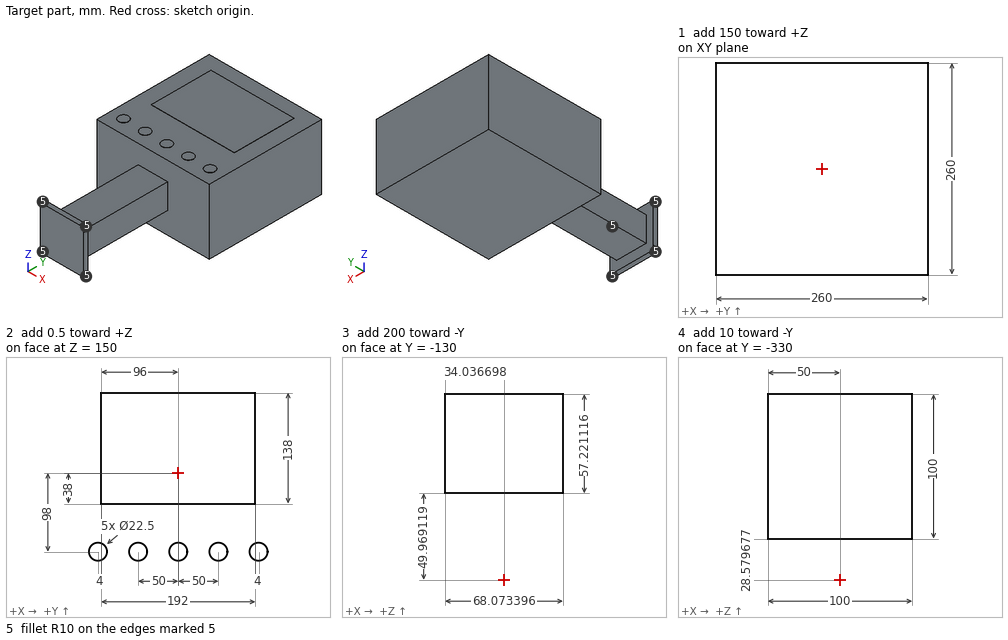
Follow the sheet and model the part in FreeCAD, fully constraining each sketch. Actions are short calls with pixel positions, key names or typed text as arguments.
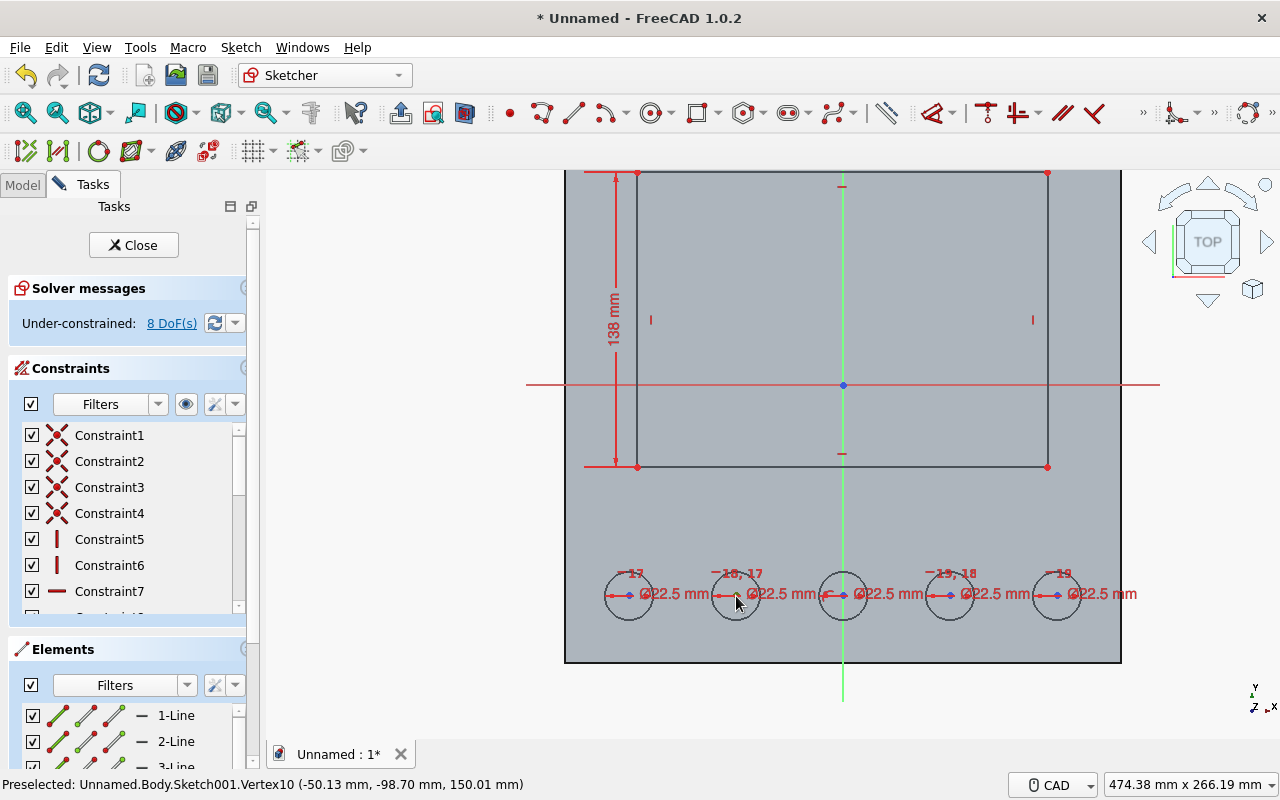
click(843, 596)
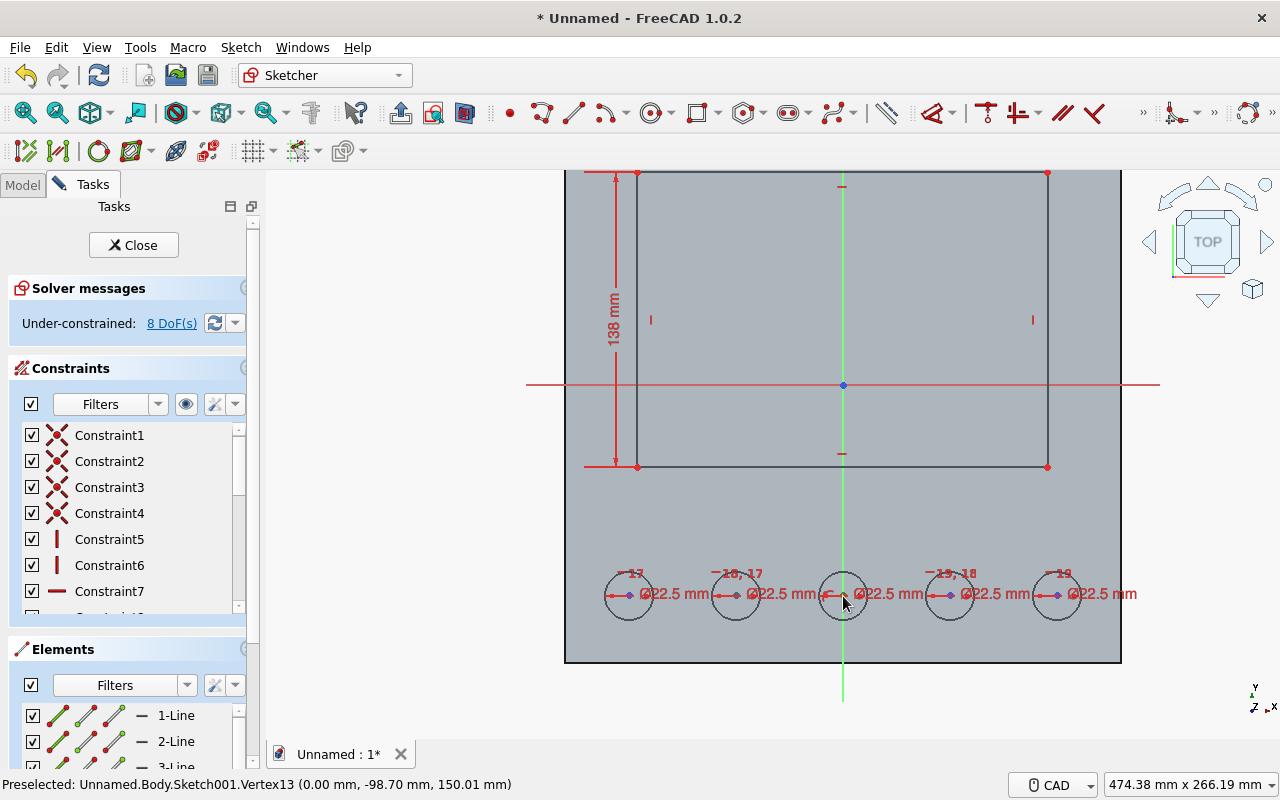
key(h)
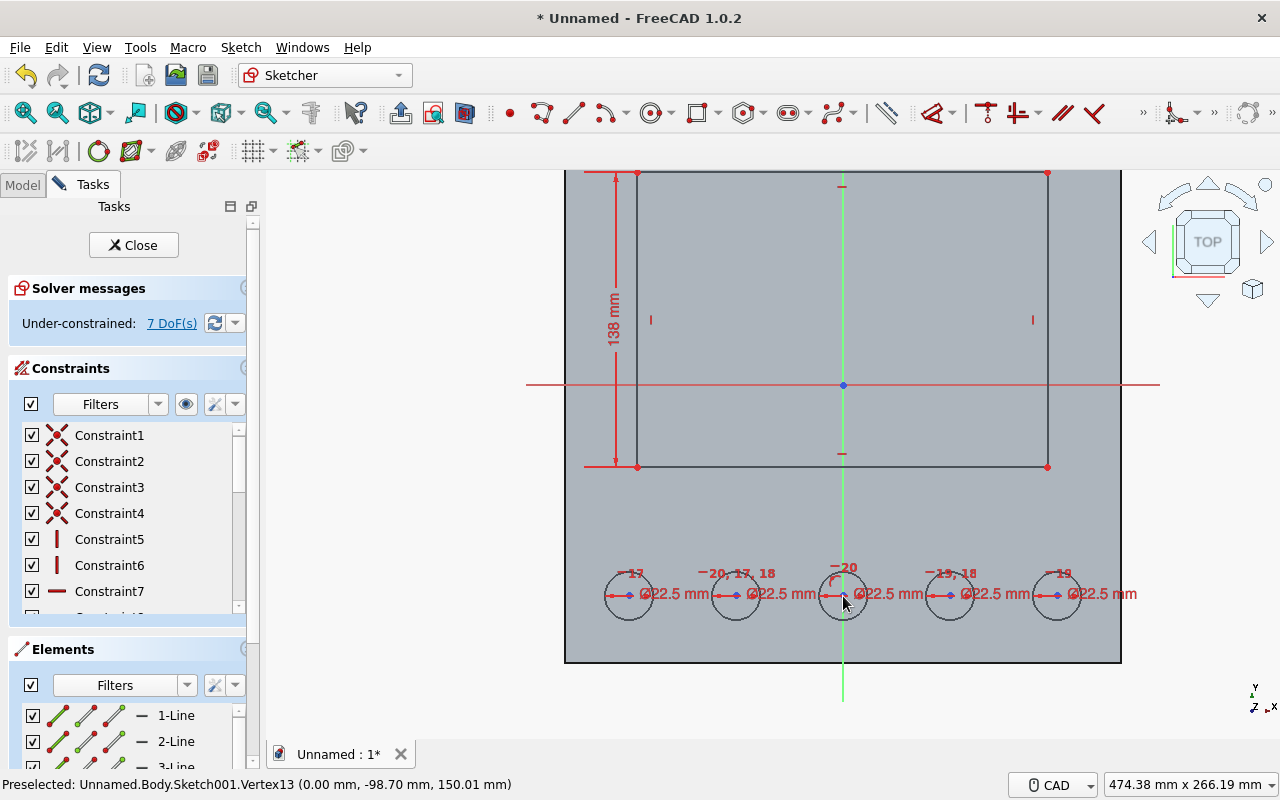
click(629, 596)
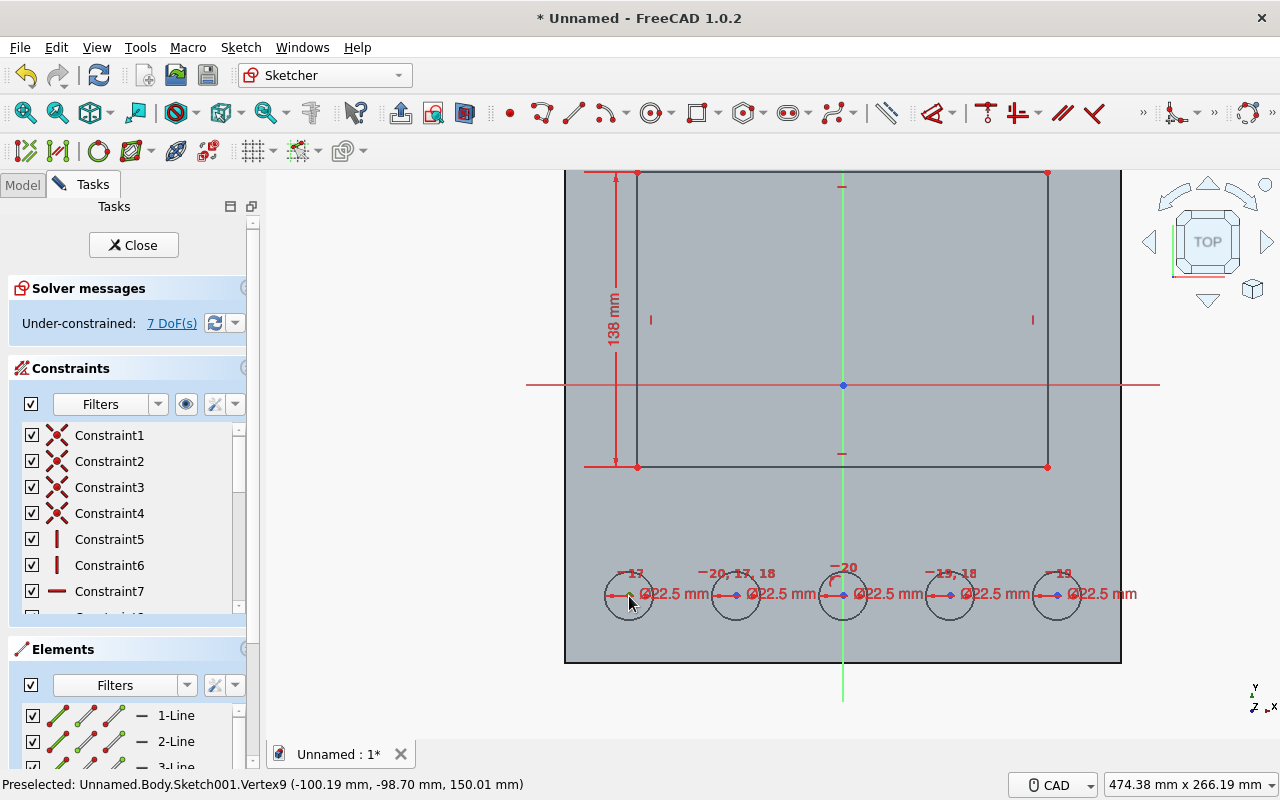
click(954, 114)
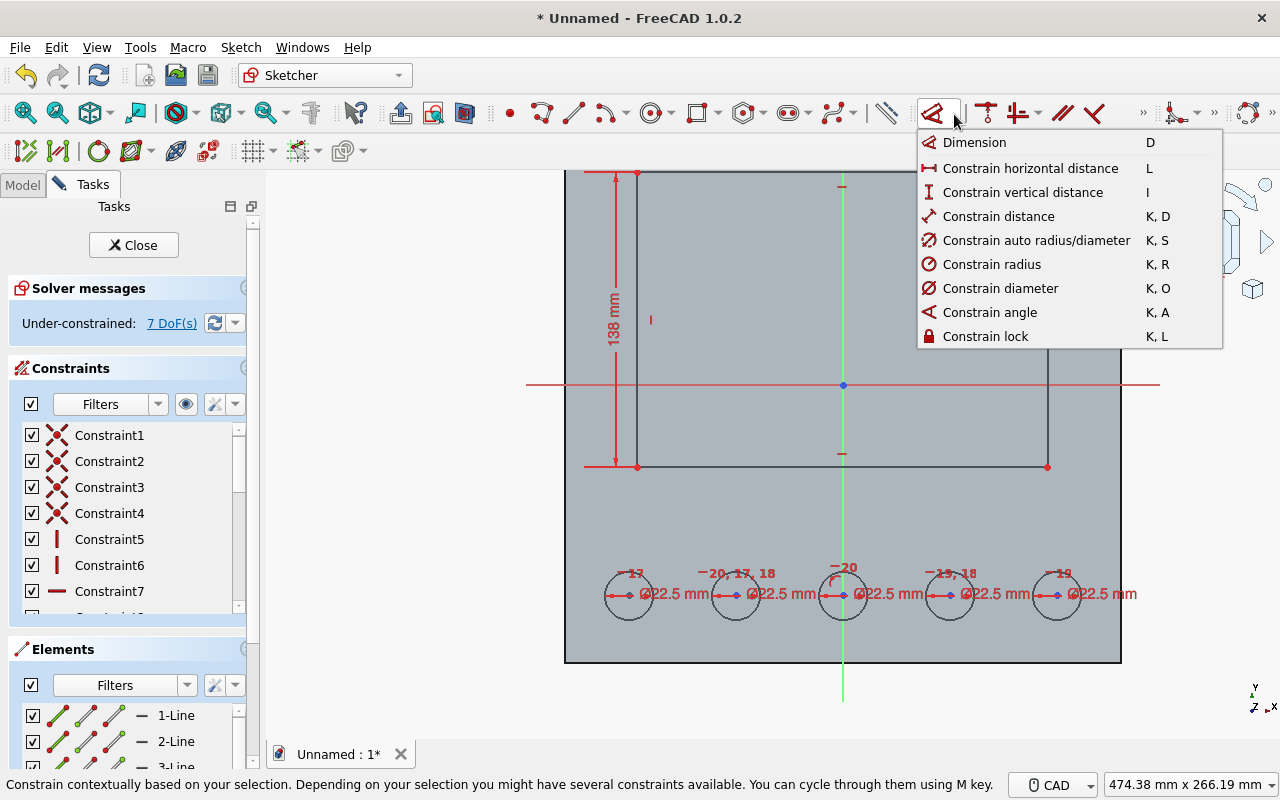
click(1070, 192)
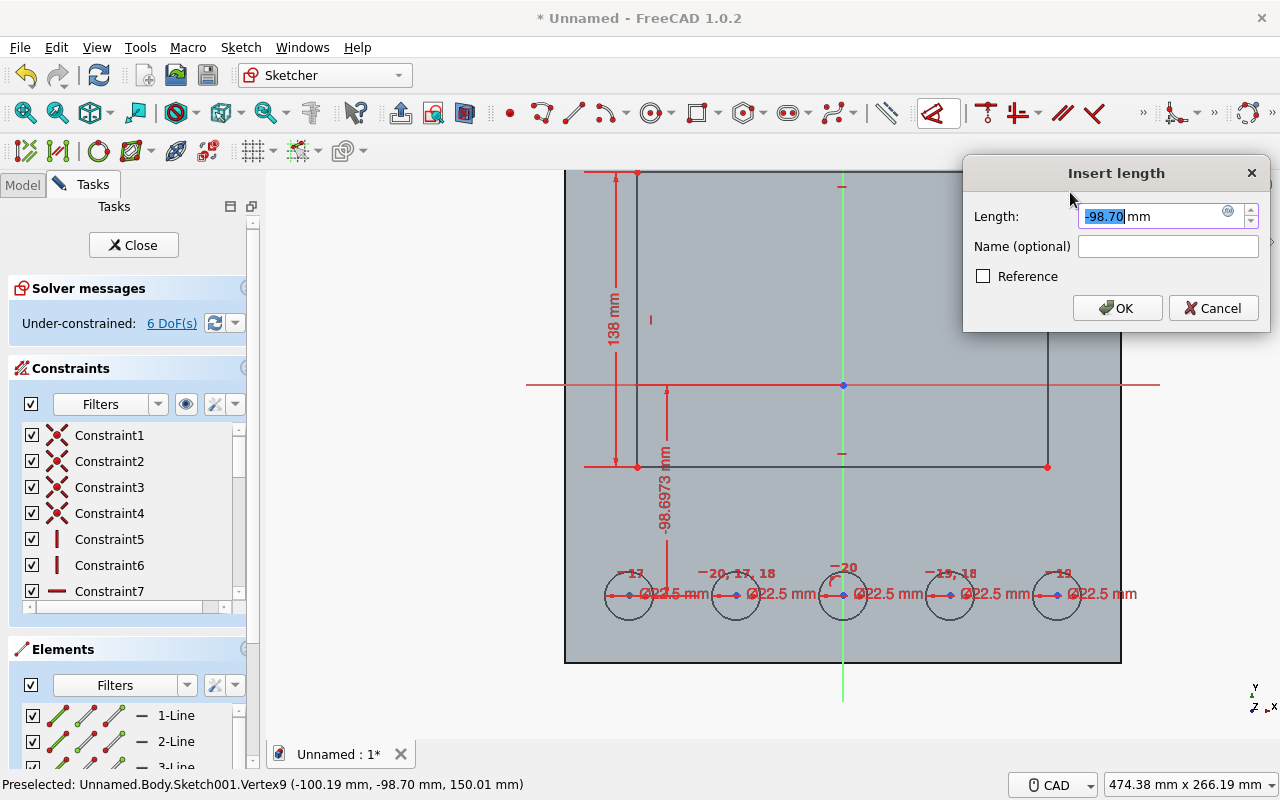
text(-98)
key(Return)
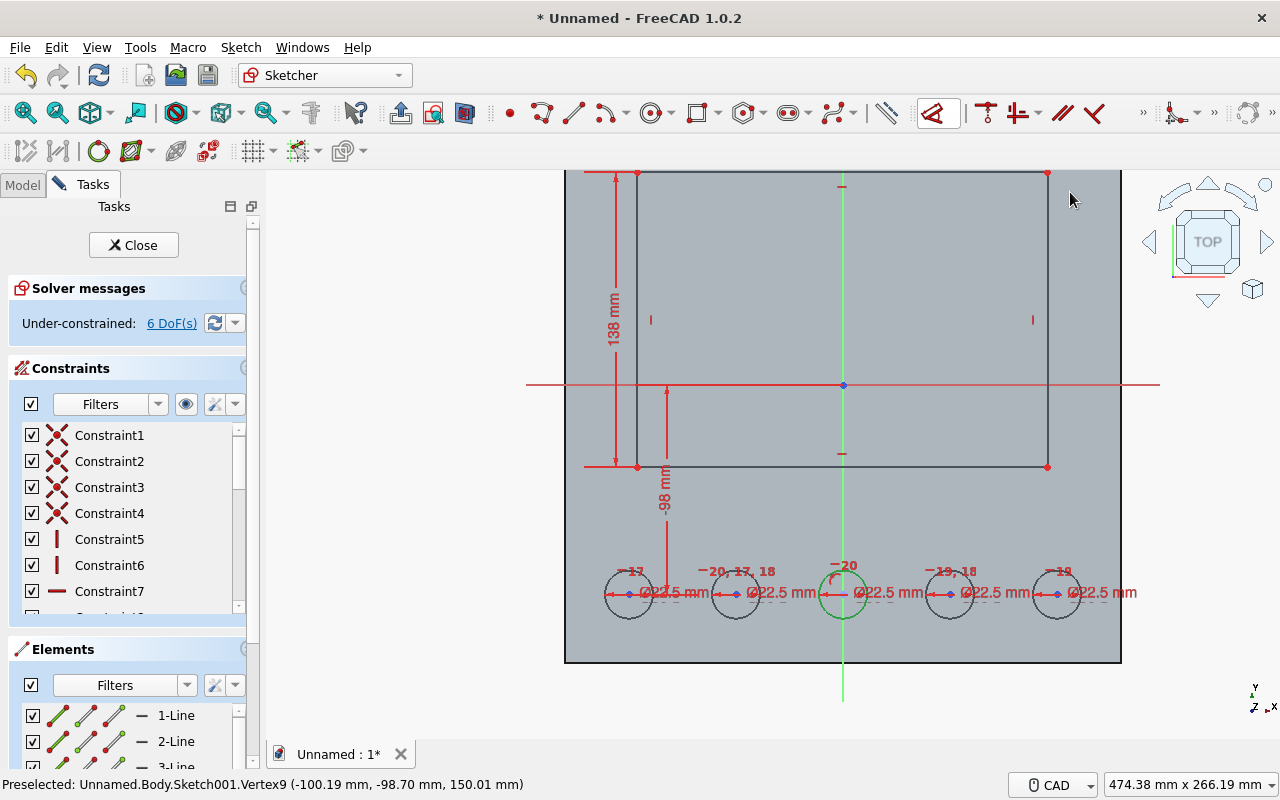
click(736, 595)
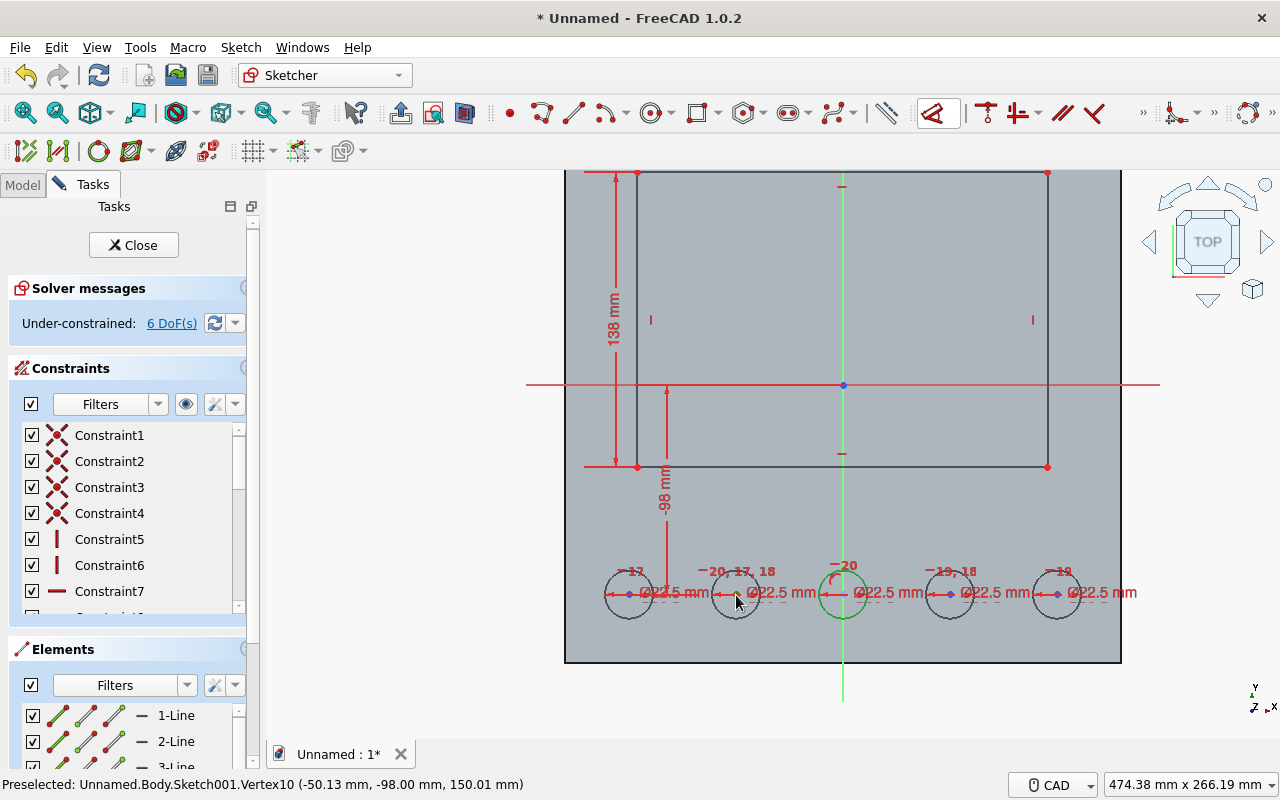
key(l)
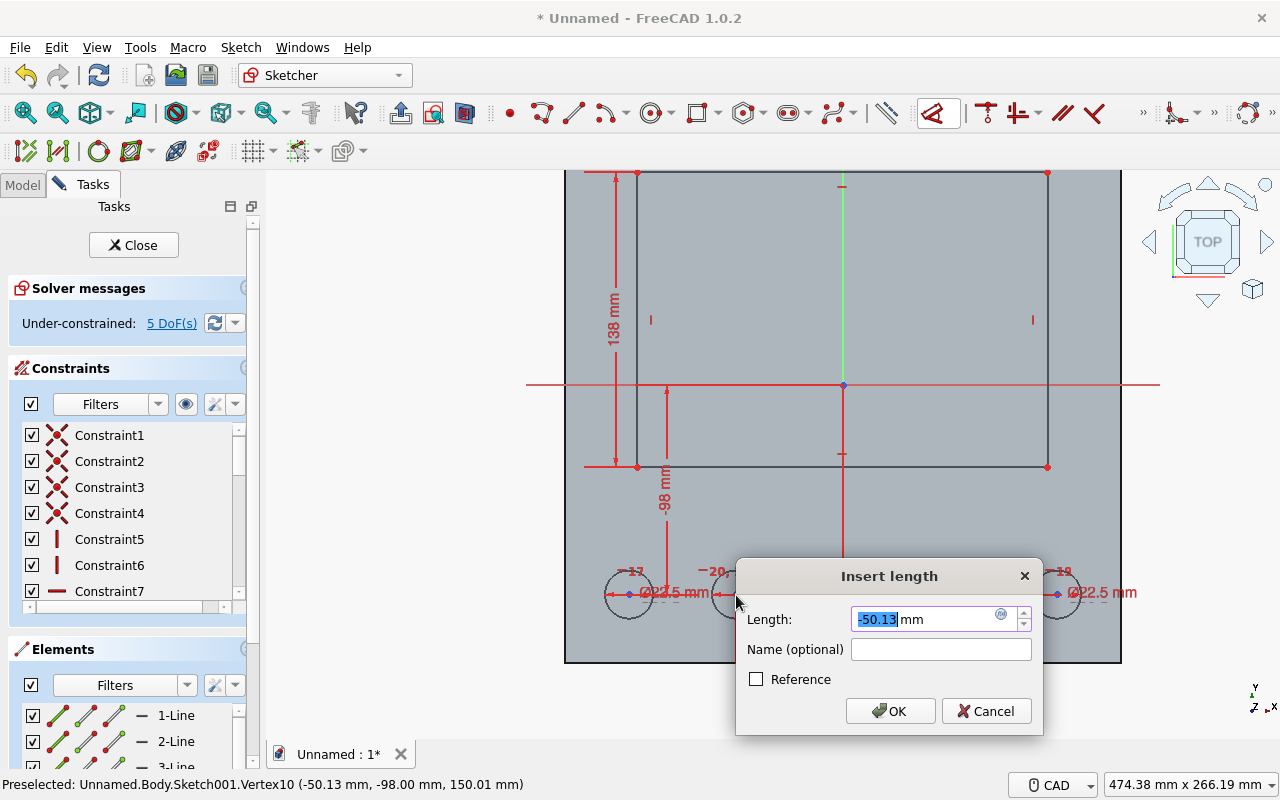
text(-50)
key(Return)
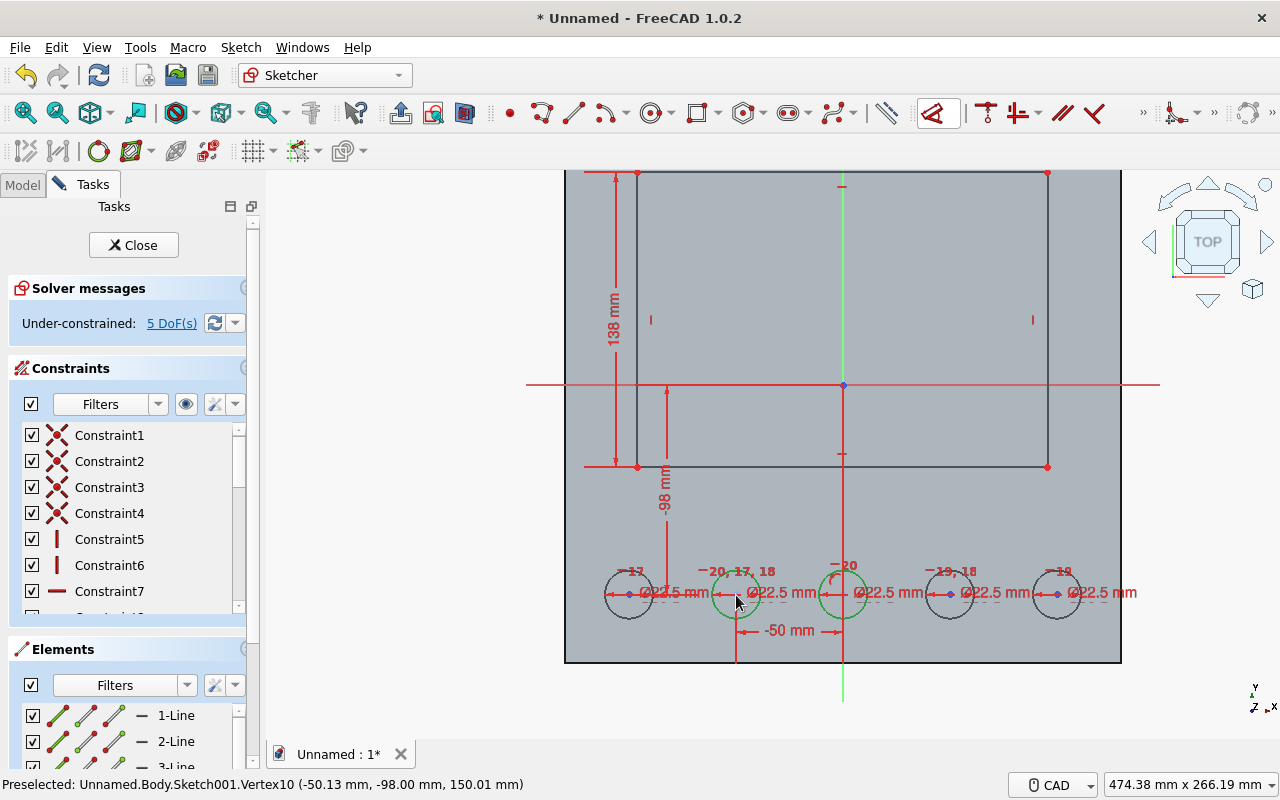
click(950, 595)